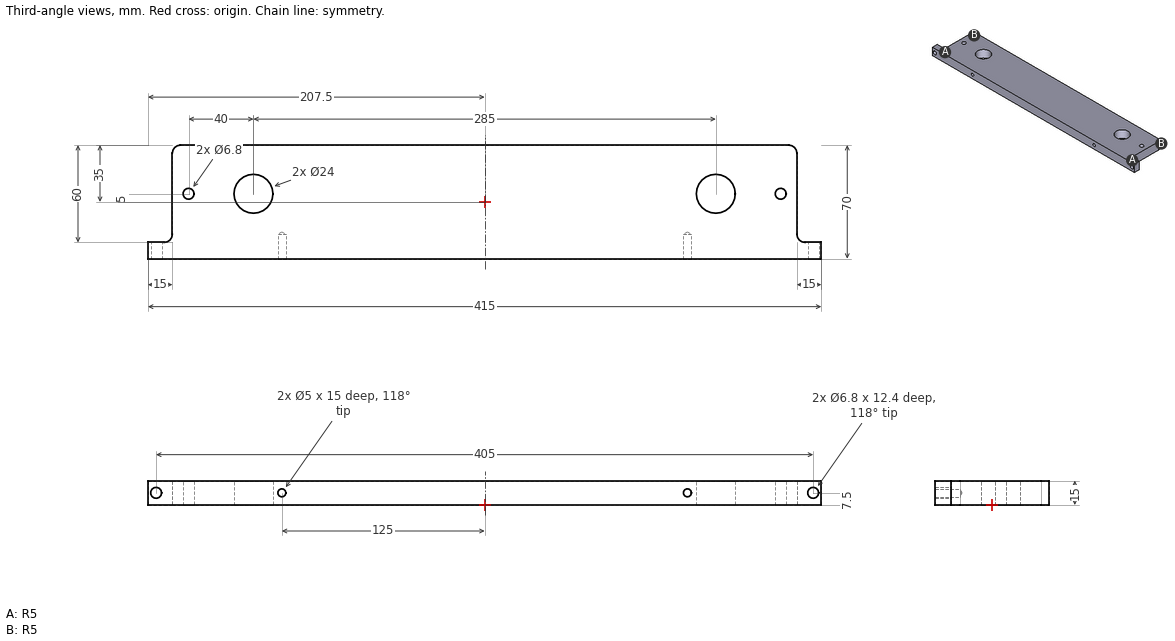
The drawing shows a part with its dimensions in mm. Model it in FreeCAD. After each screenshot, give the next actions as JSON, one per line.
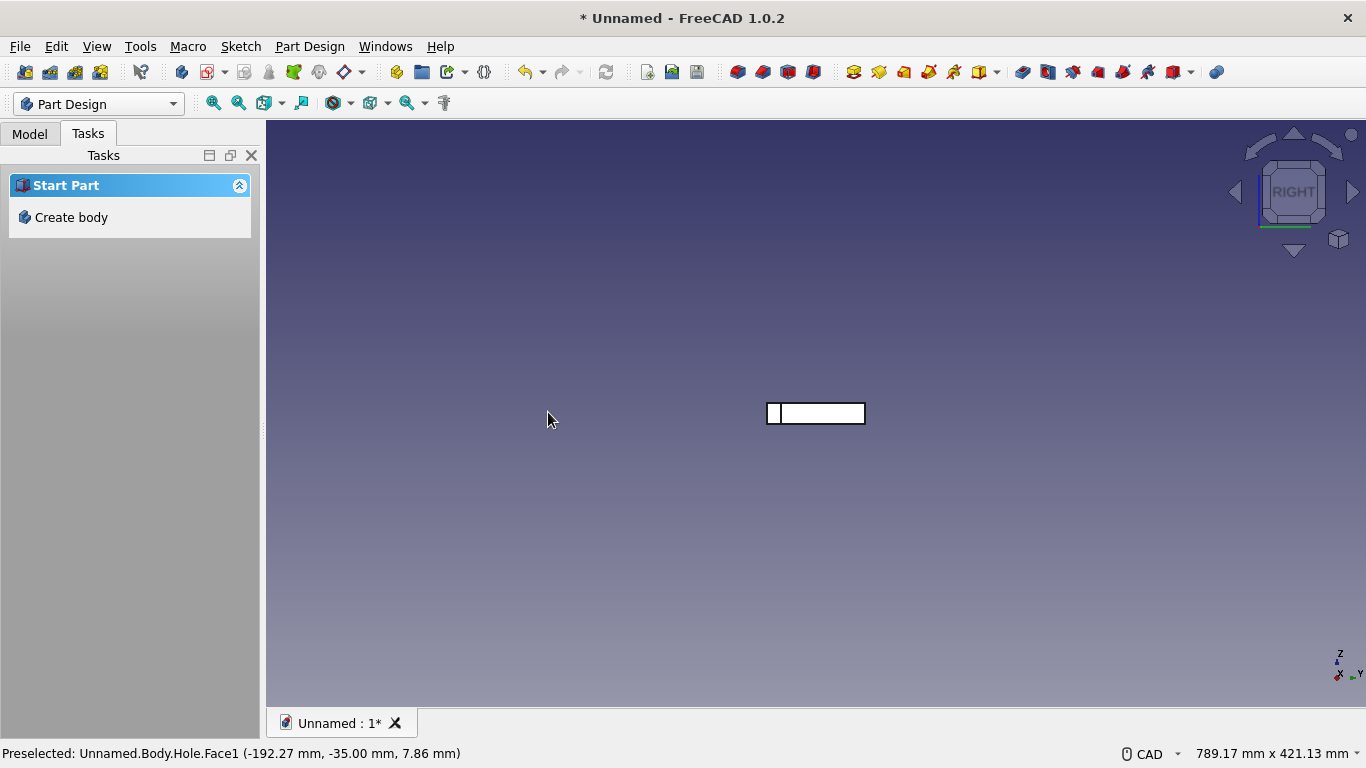
{"action": "scroll", "coordinate": [781, 412], "scroll_direction": "up", "scroll_amount": 4}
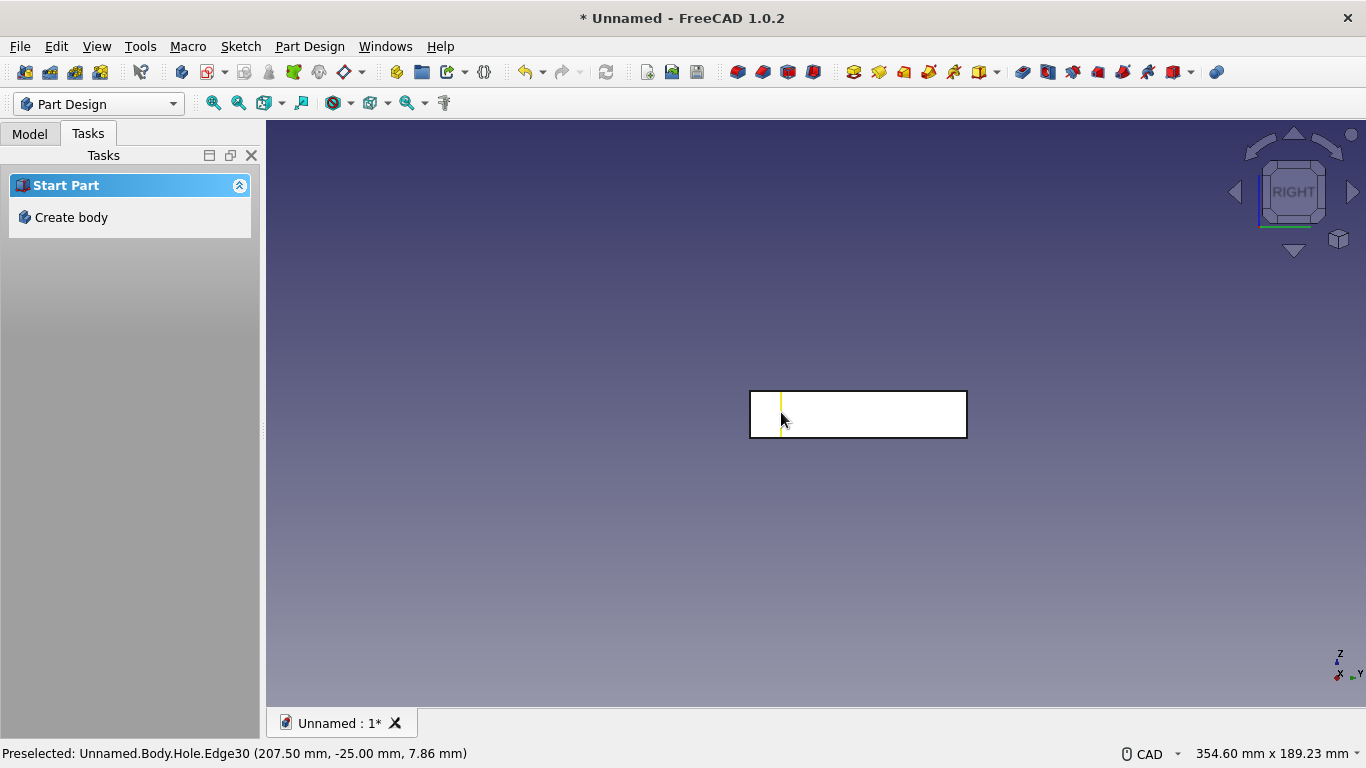
{"action": "key", "text": "v f"}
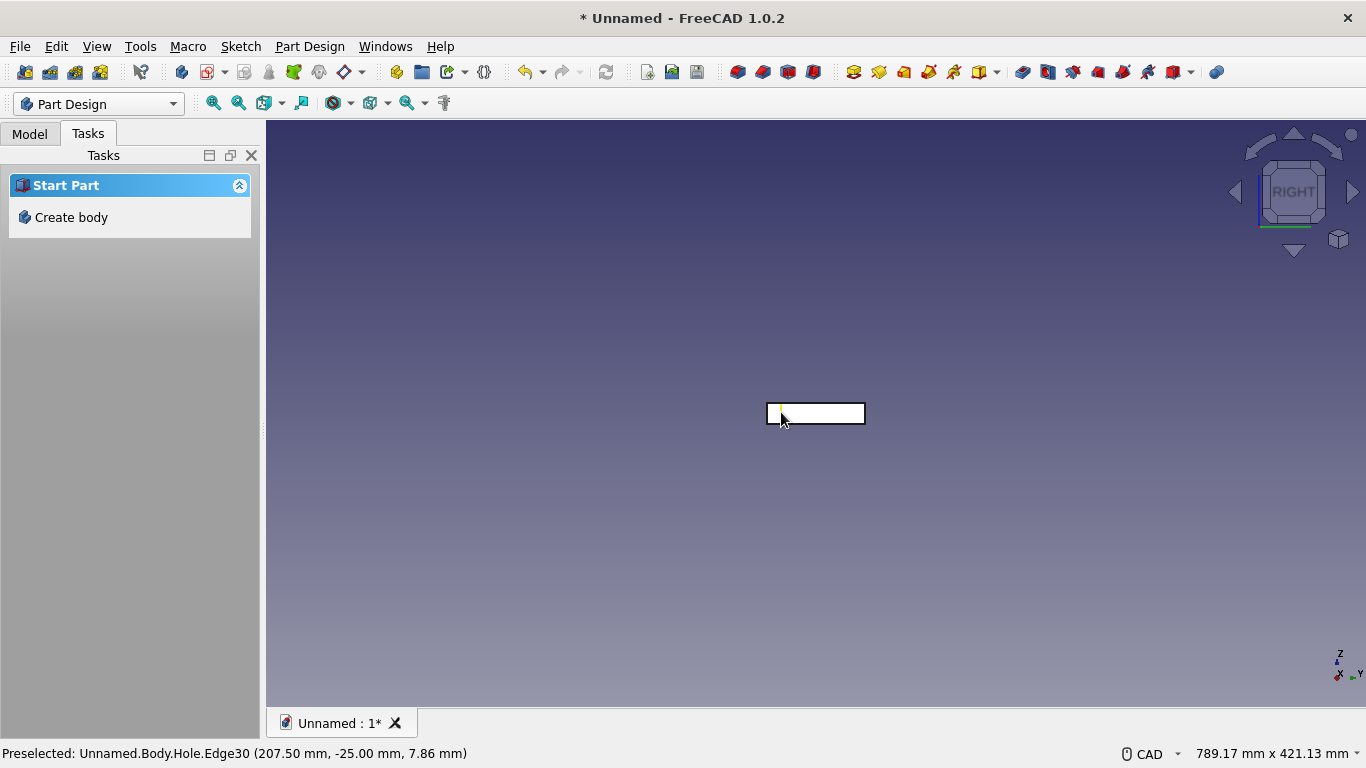
{"action": "key", "text": "5"}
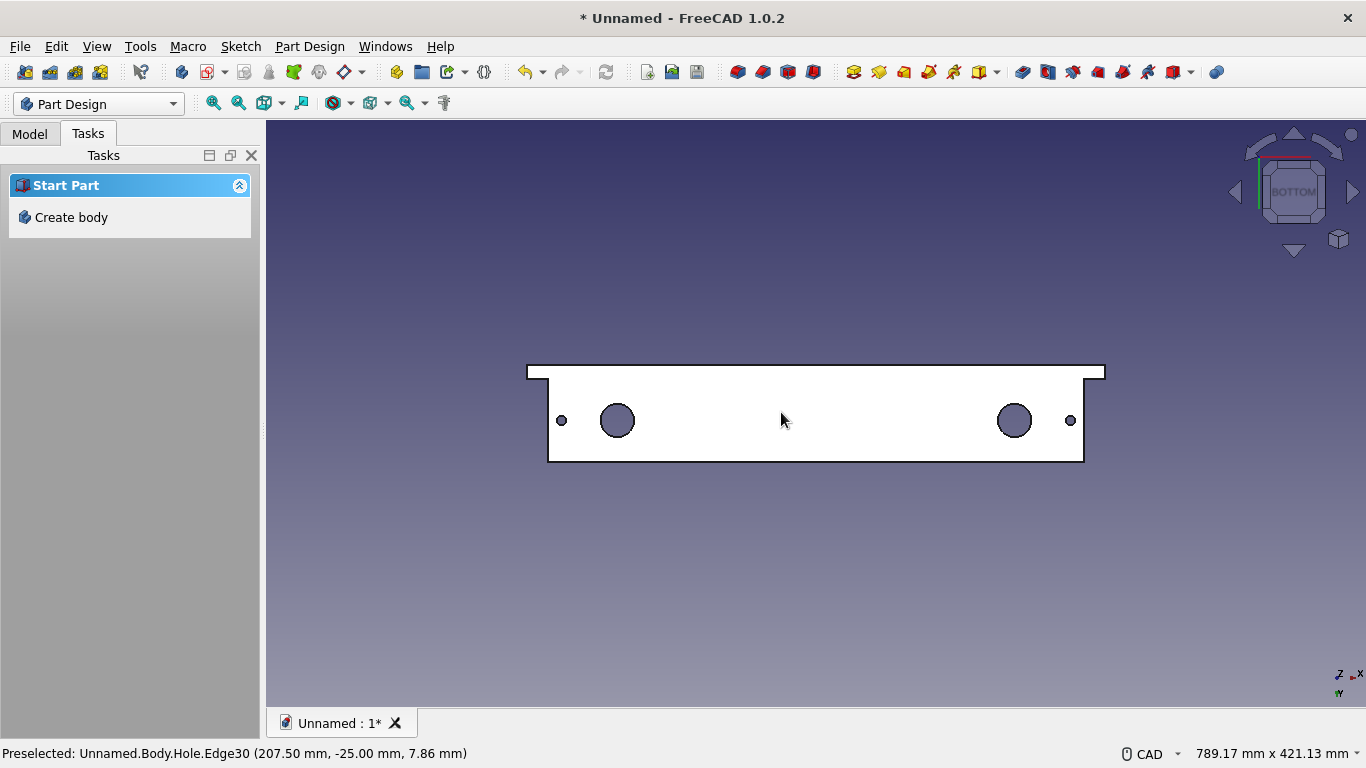
{"action": "scroll", "coordinate": [548, 378], "scroll_direction": "up", "scroll_amount": 4}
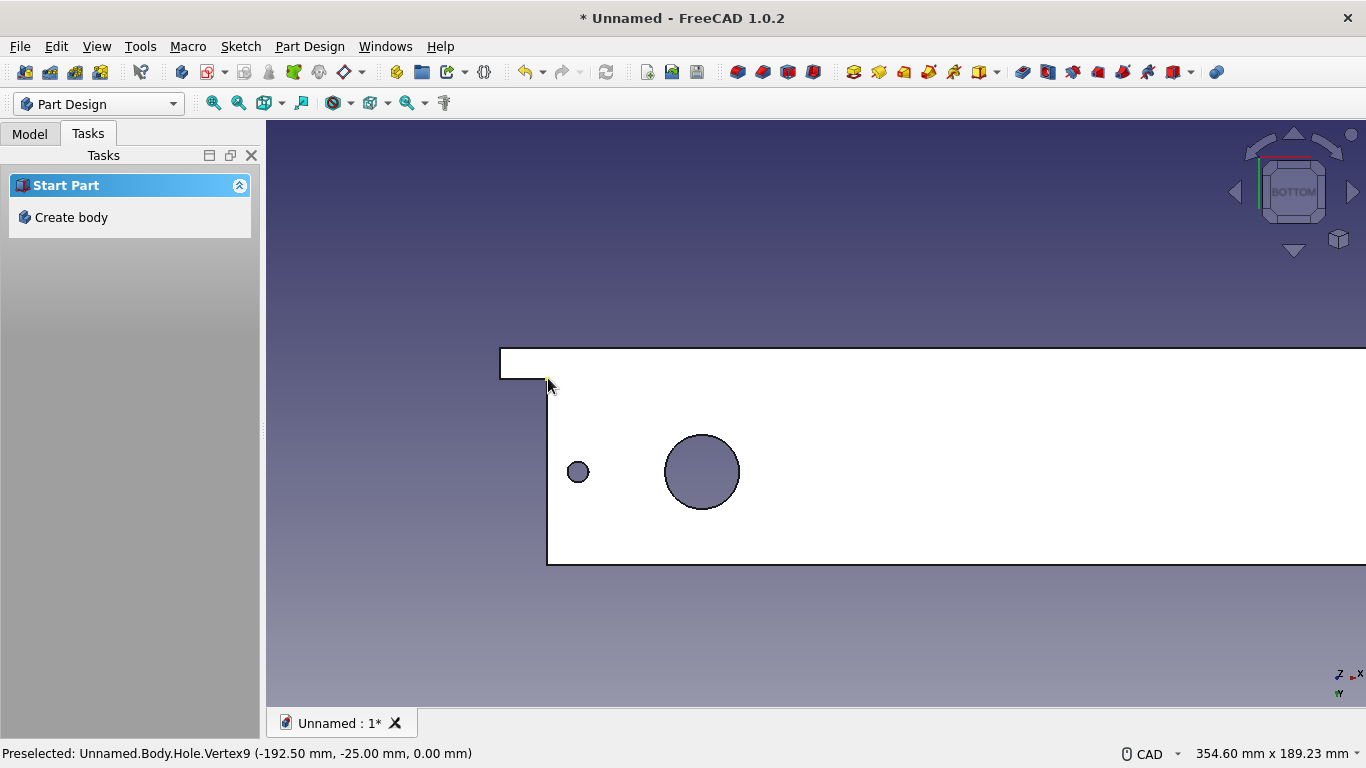
{"action": "key", "text": "v f"}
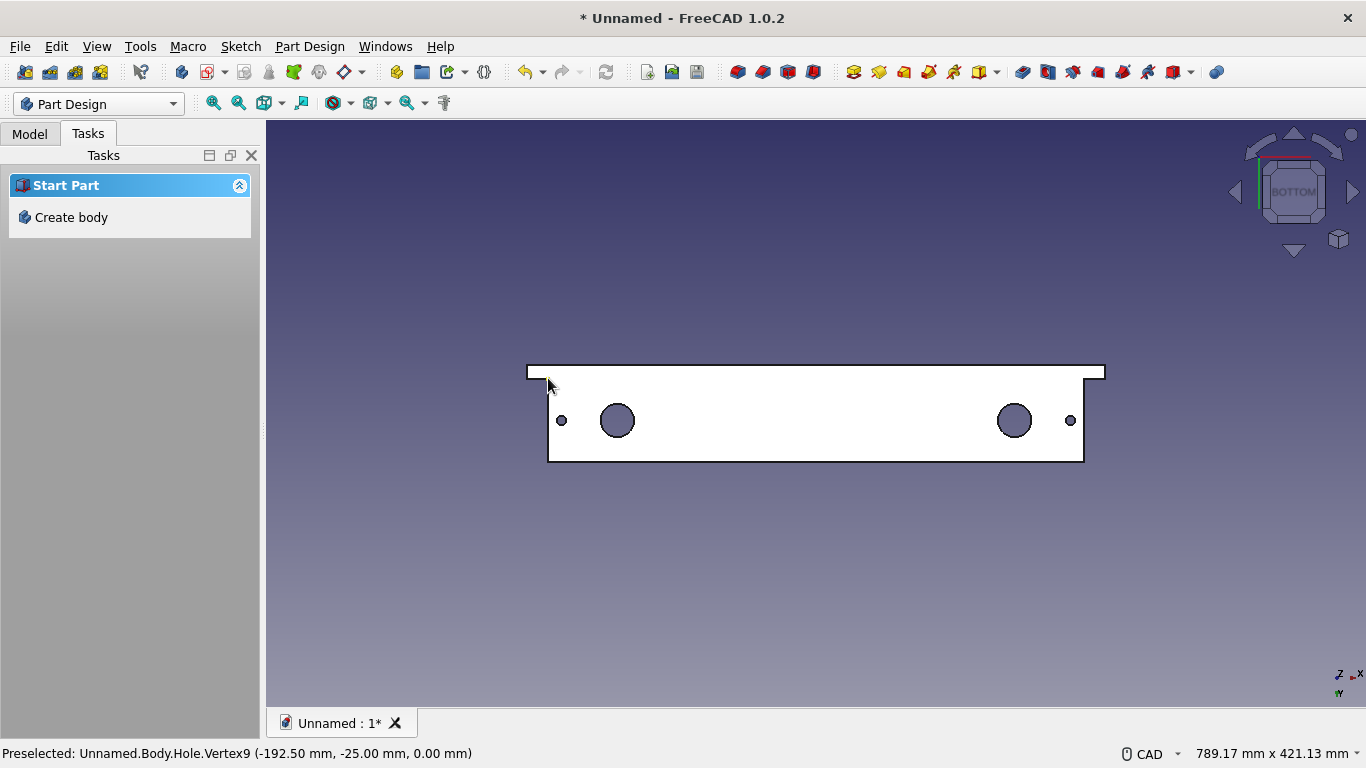
{"action": "key", "text": "4"}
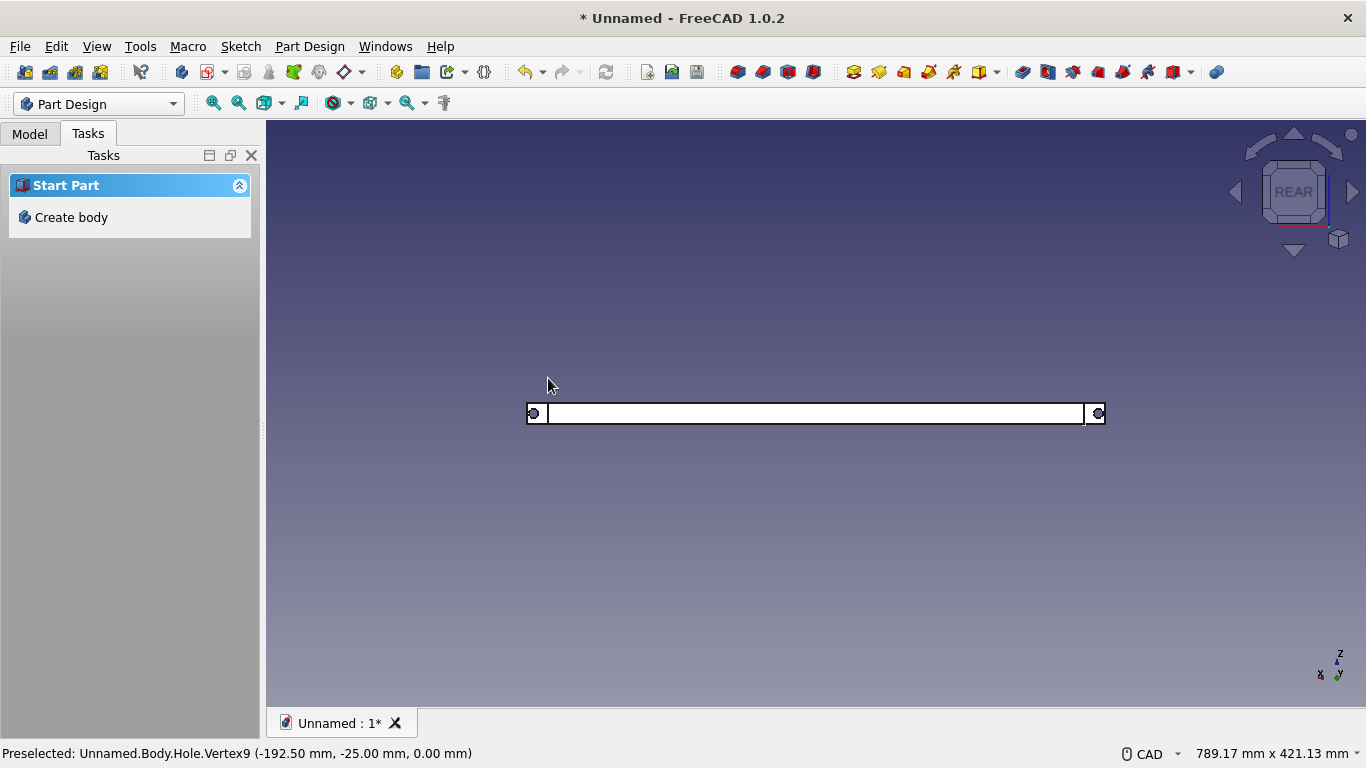
{"action": "scroll", "coordinate": [1084, 412], "scroll_direction": "up", "scroll_amount": 4}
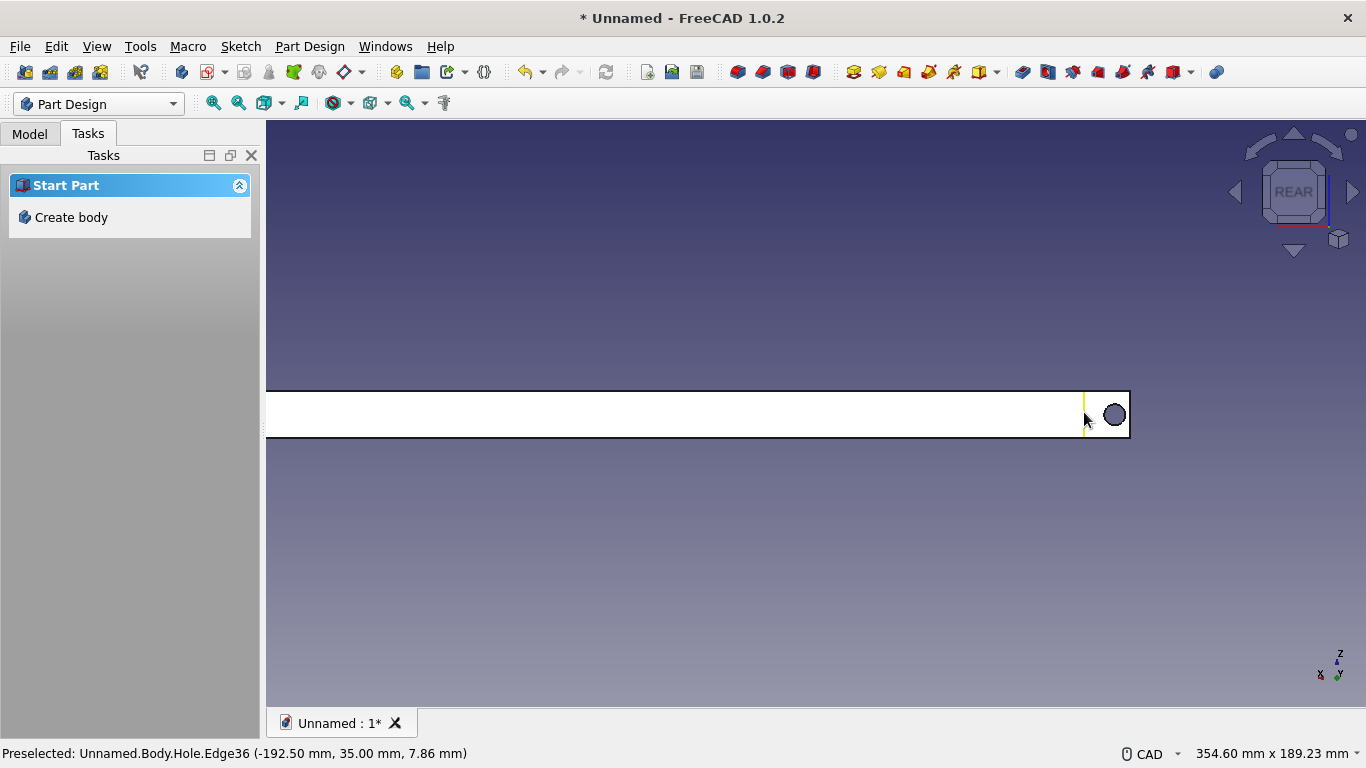
{"action": "key", "text": "v f"}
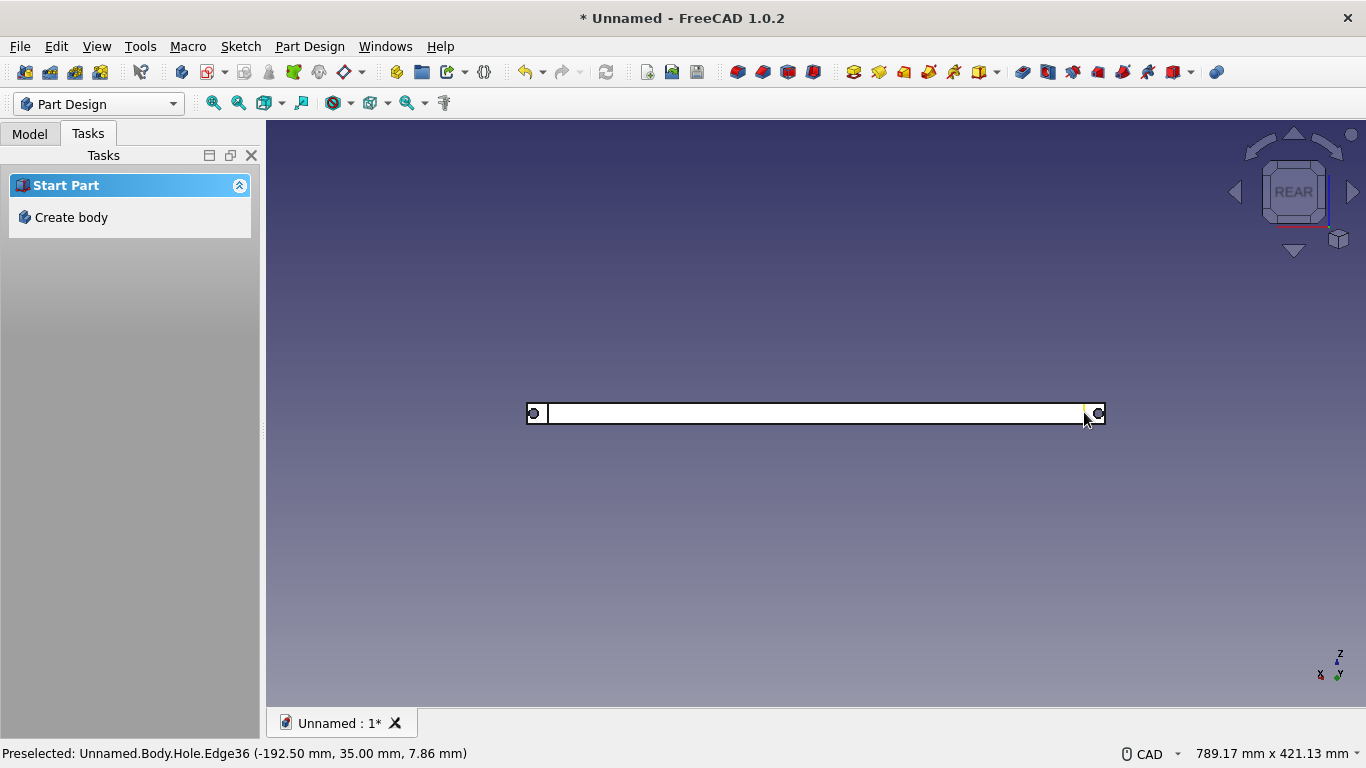
{"action": "key", "text": "6"}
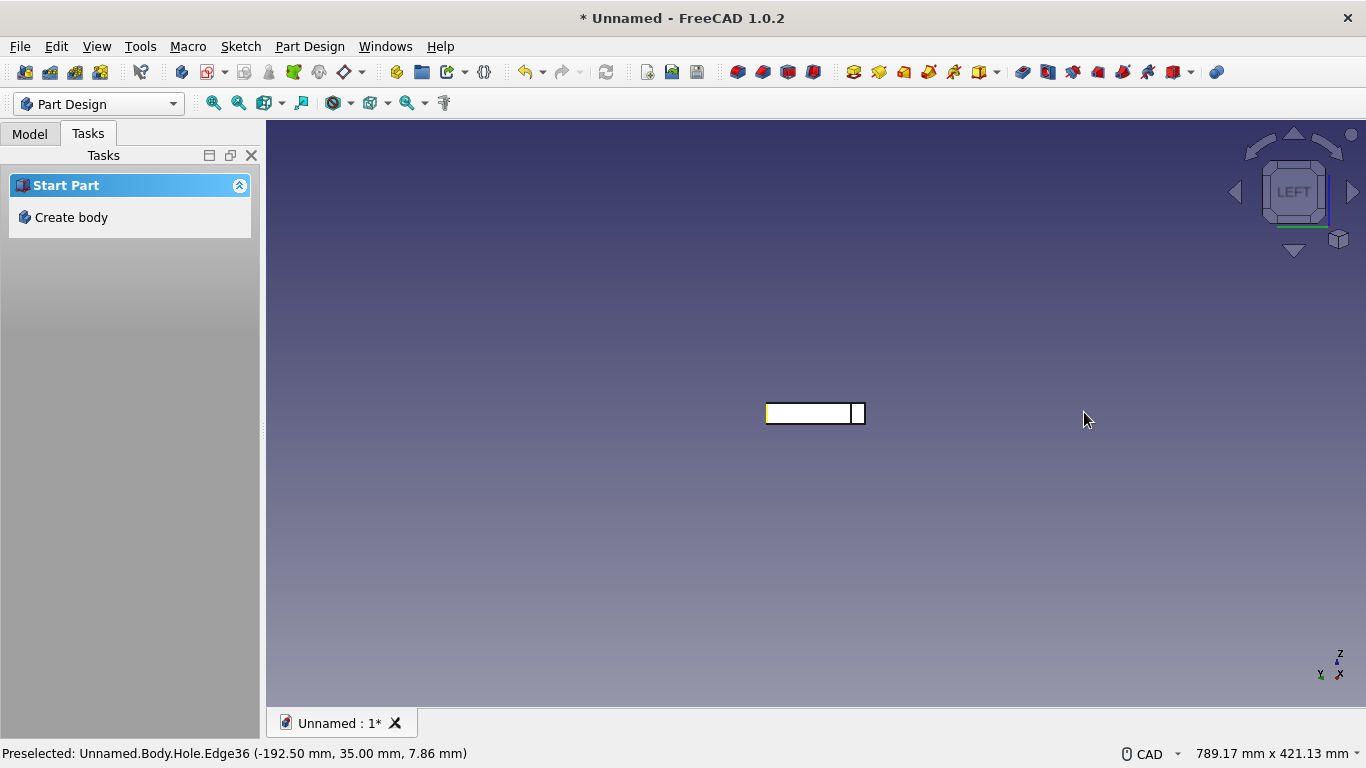
{"action": "left_click", "coordinate": [214, 104]}